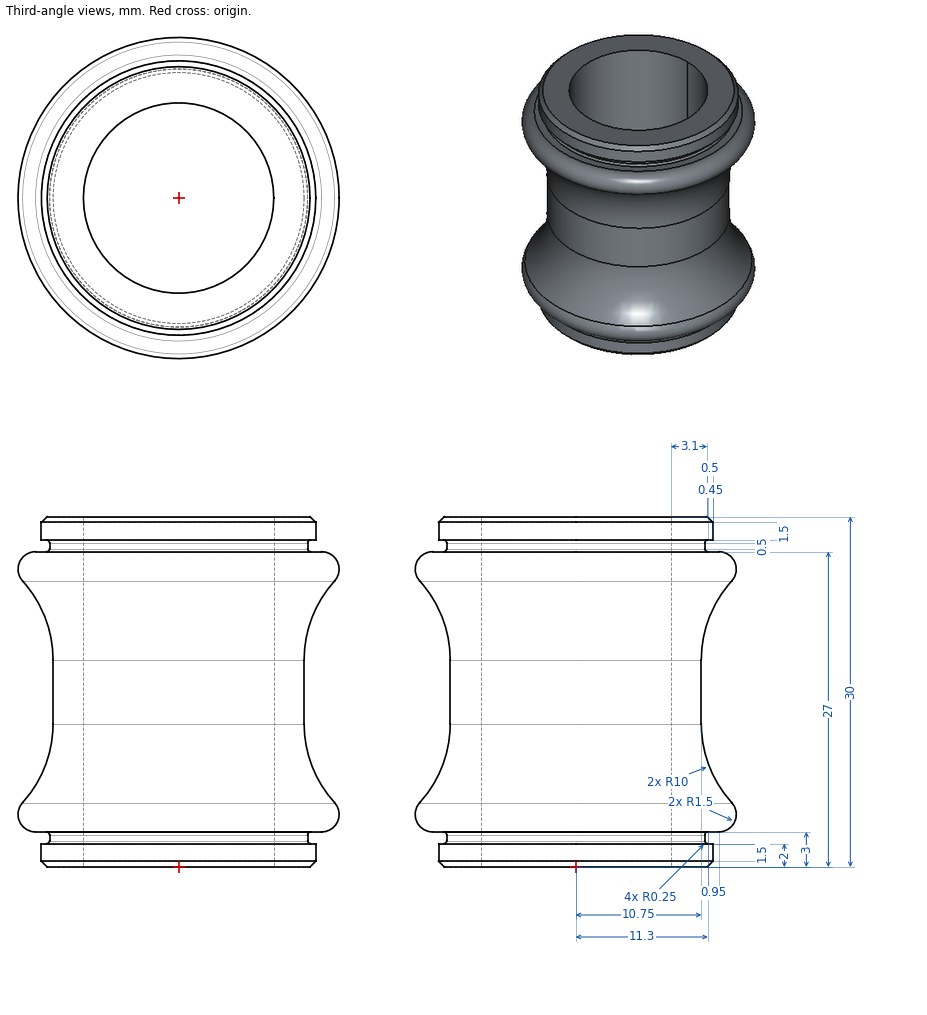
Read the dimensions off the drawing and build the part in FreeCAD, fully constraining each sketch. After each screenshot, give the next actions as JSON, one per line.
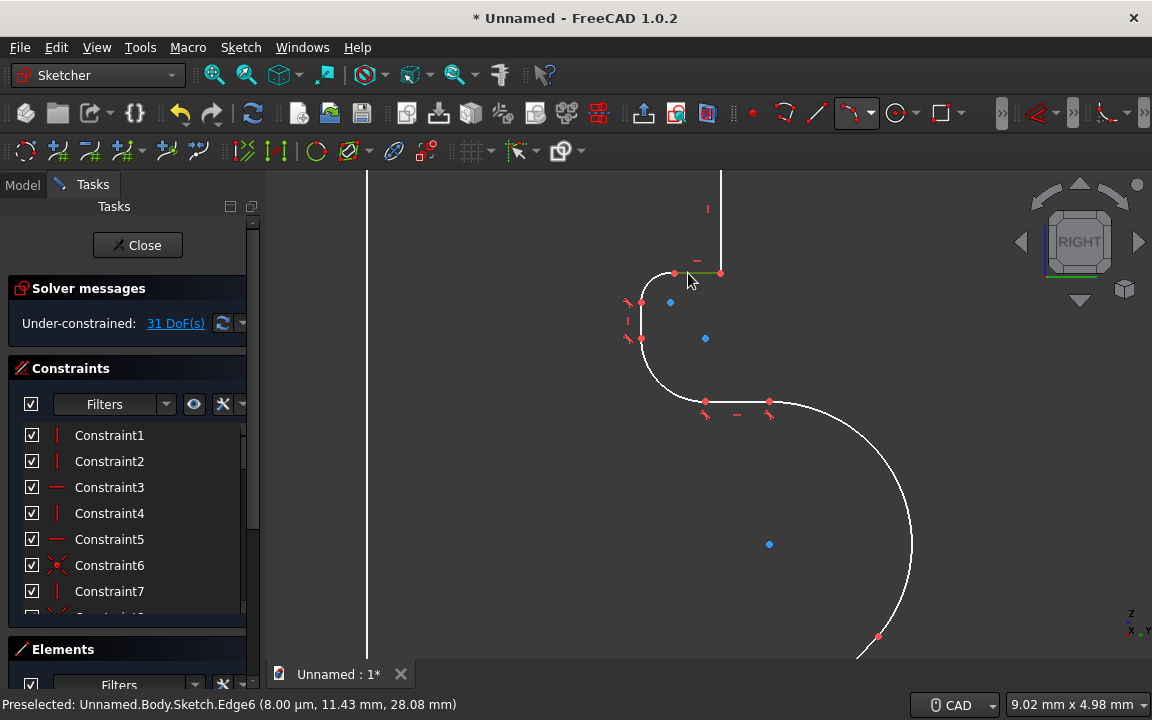
{"action": "left_click", "coordinate": [659, 275]}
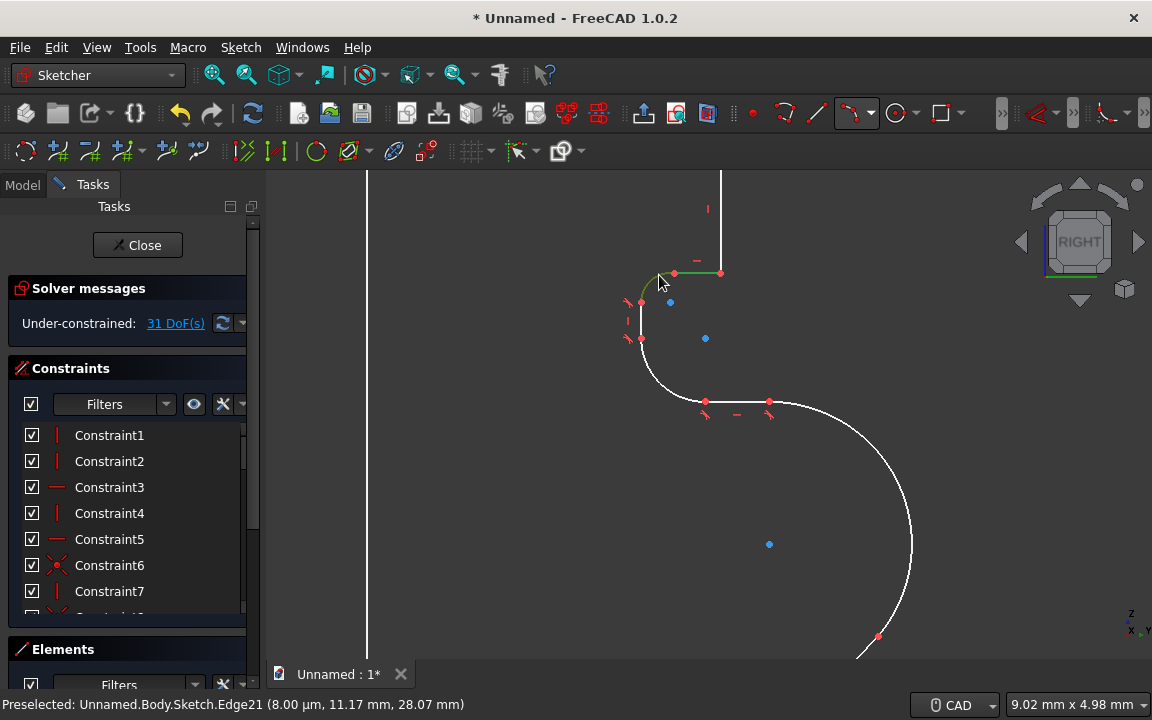
{"action": "key", "text": "t"}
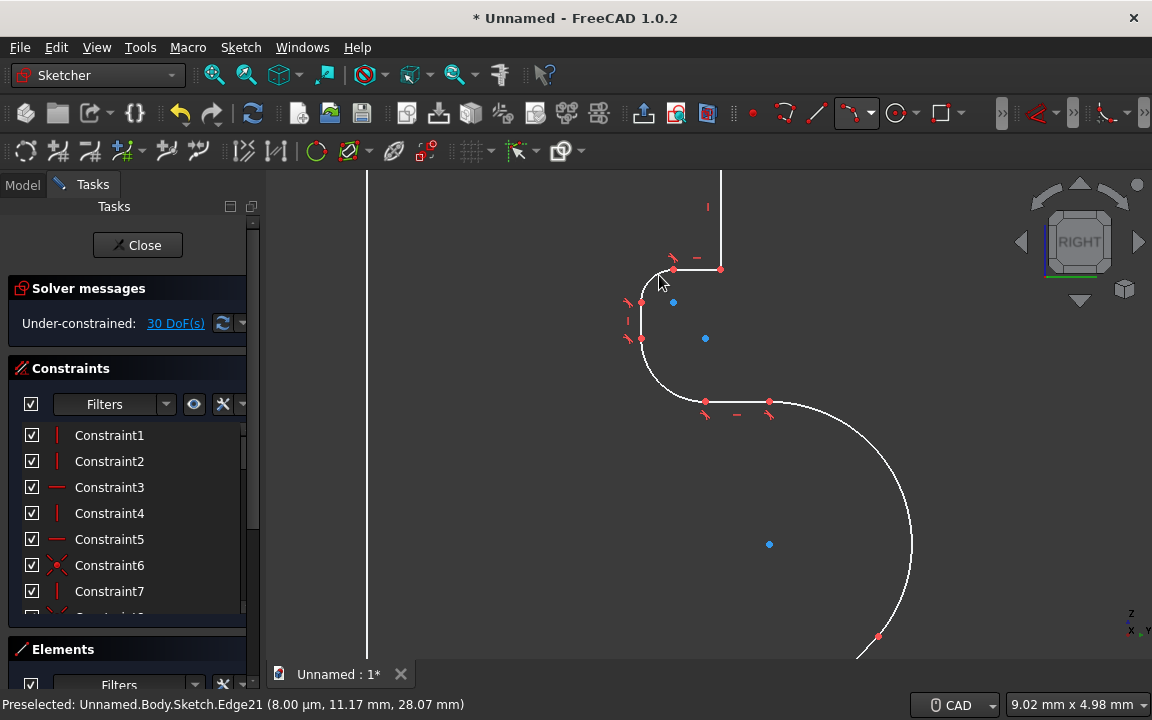
{"action": "scroll", "coordinate": [691, 272], "scroll_direction": "down", "scroll_amount": 11}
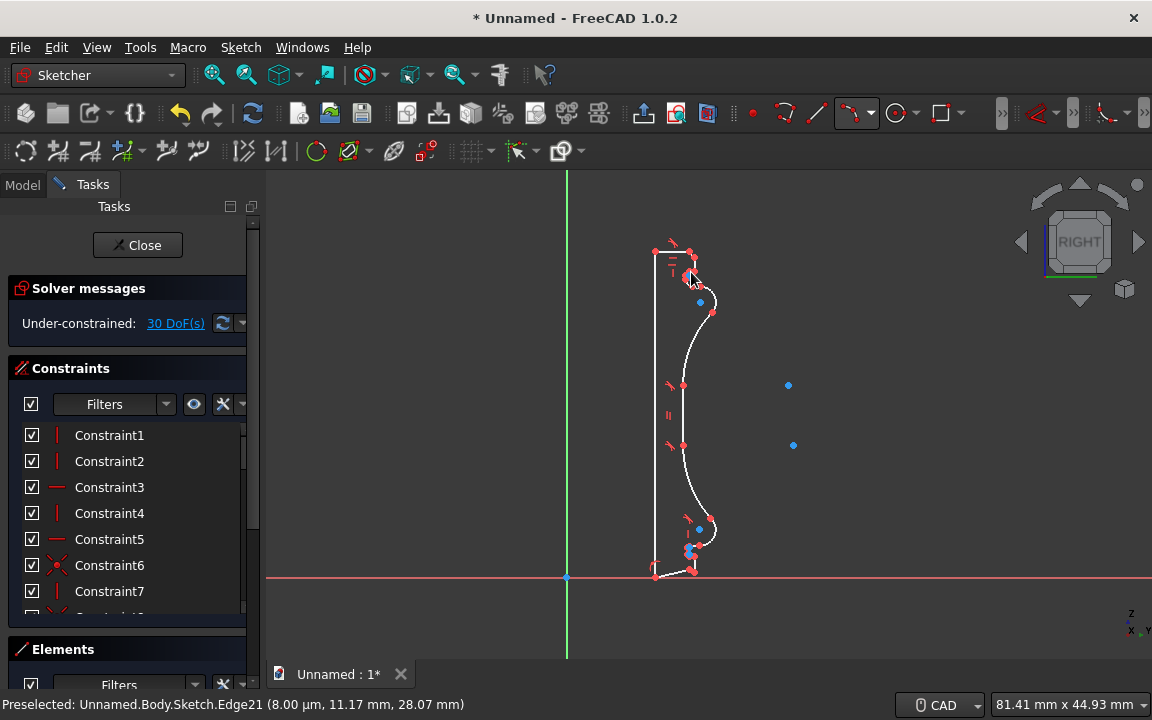
{"action": "scroll", "coordinate": [693, 556], "scroll_direction": "up", "scroll_amount": 12}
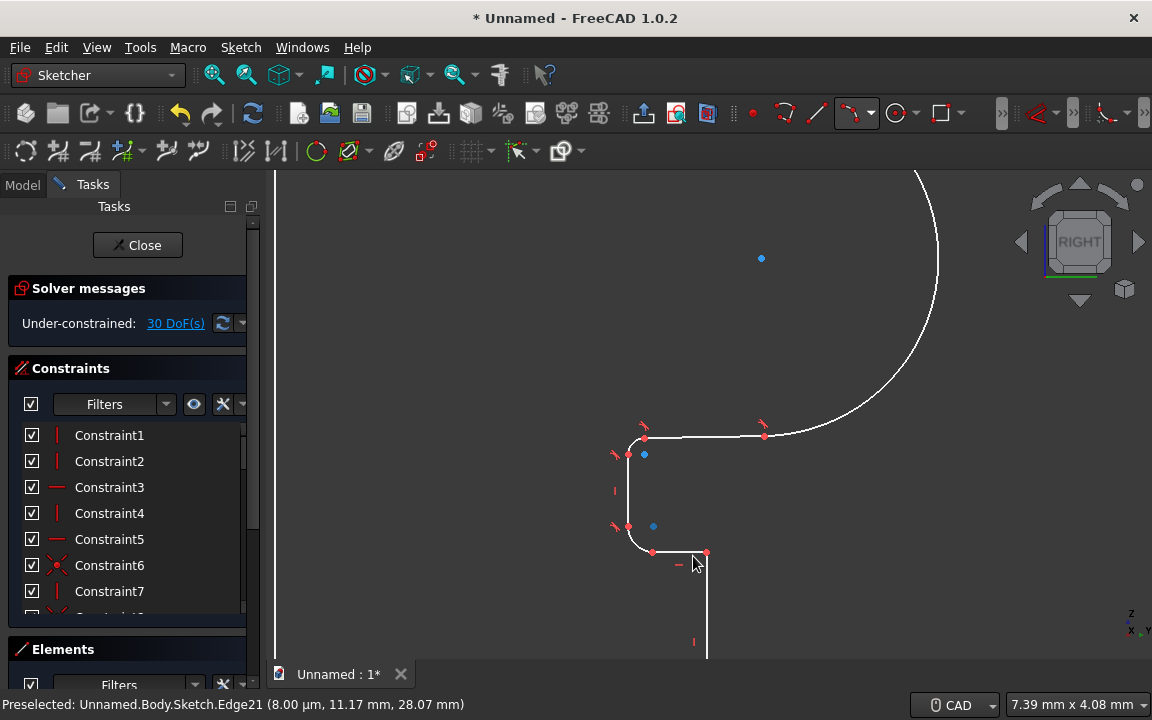
{"action": "left_click", "coordinate": [690, 552]}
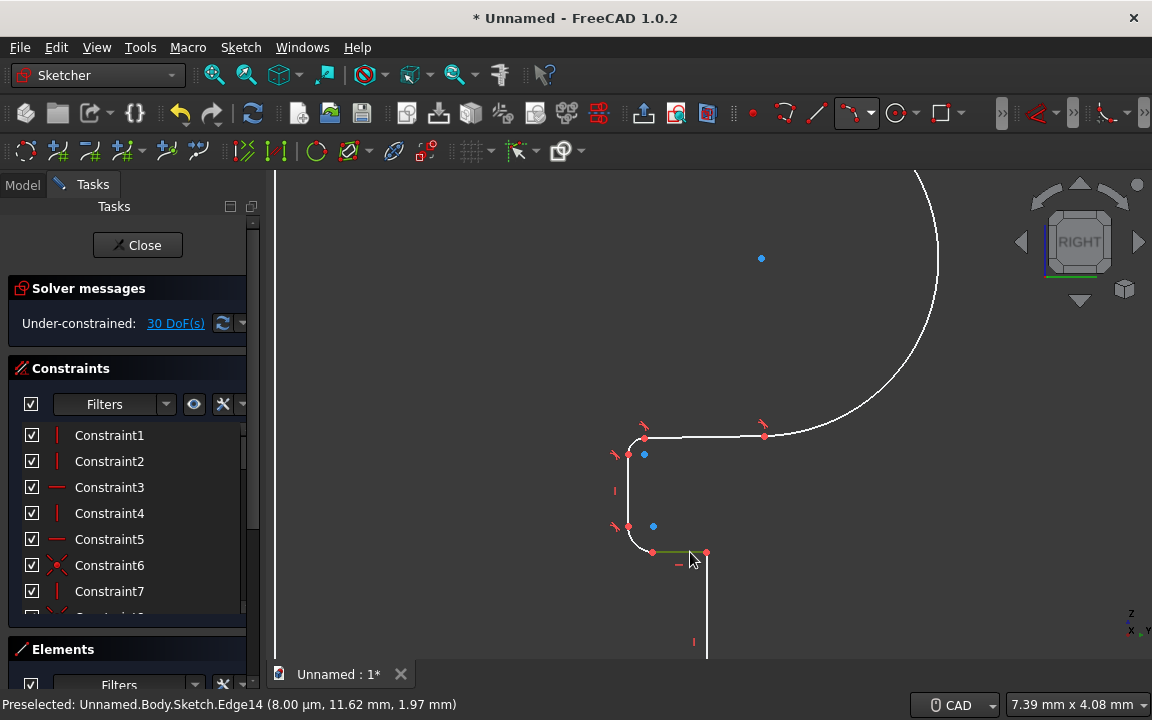
{"action": "left_click", "coordinate": [631, 538]}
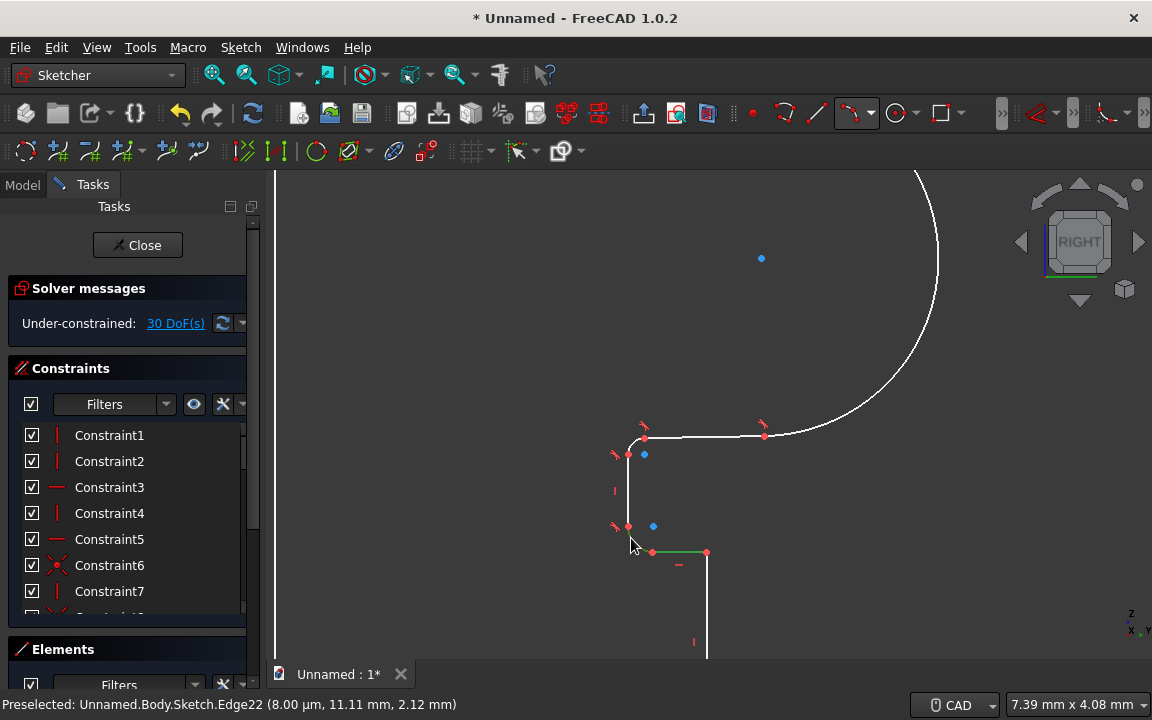
{"action": "key", "text": "t"}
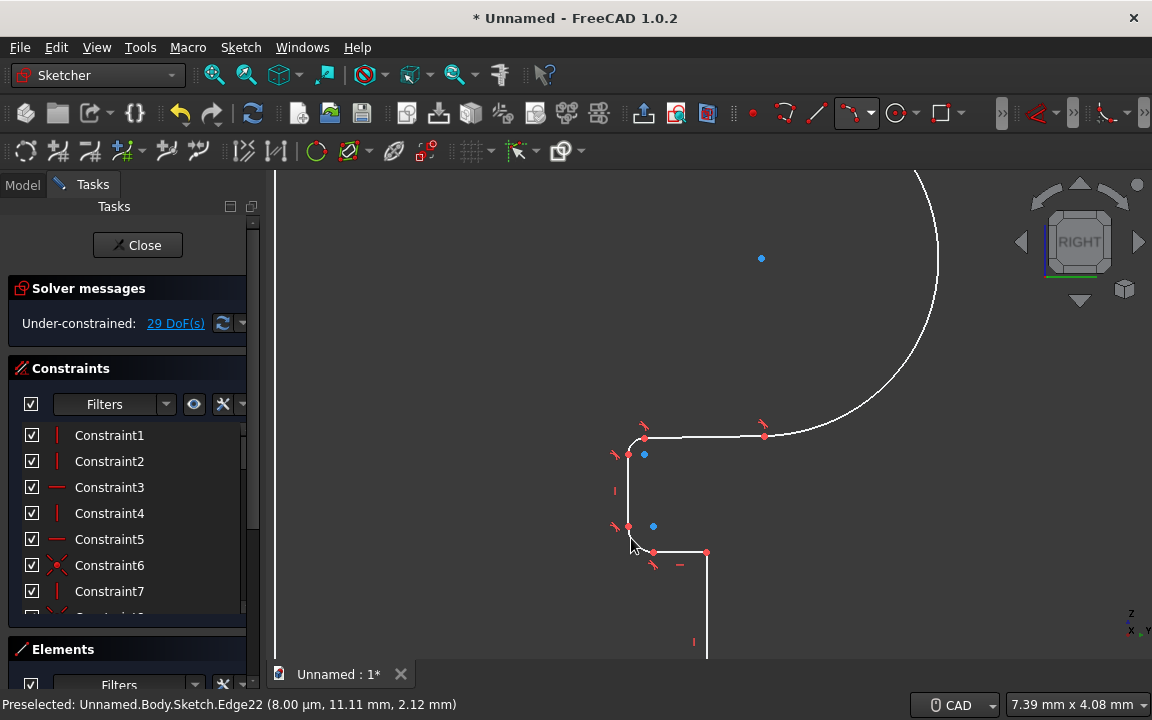
{"action": "scroll", "coordinate": [693, 557], "scroll_direction": "down", "scroll_amount": 12}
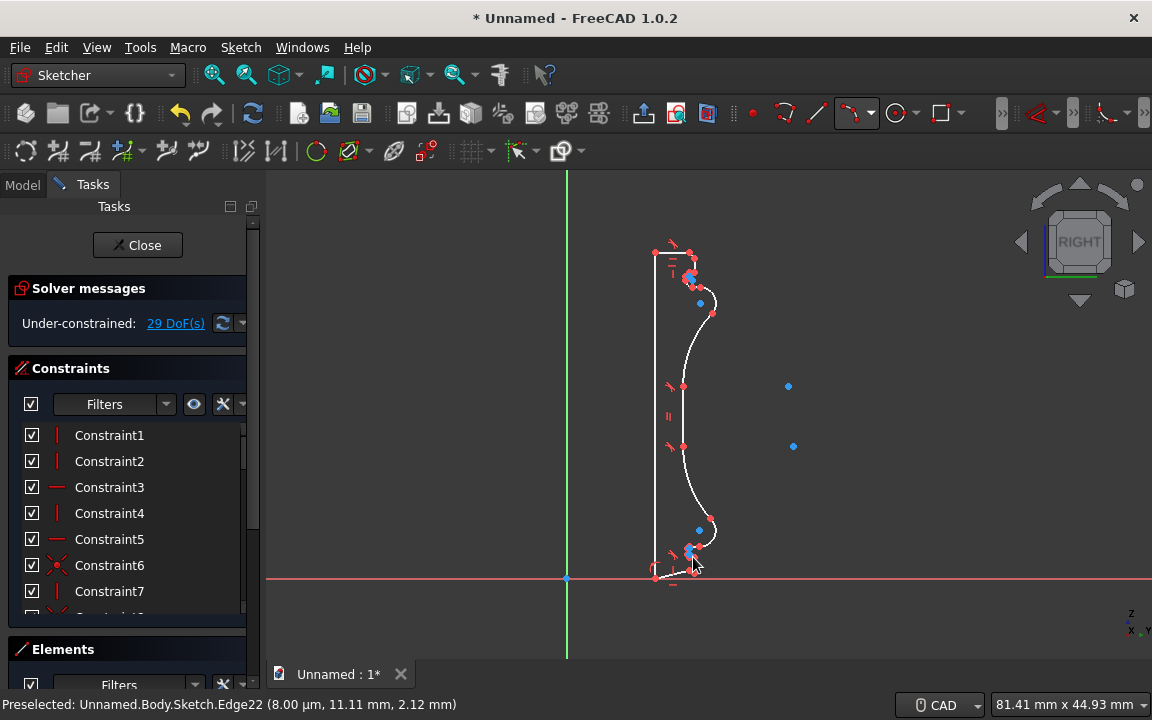
{"action": "scroll", "coordinate": [710, 543], "scroll_direction": "up", "scroll_amount": 2}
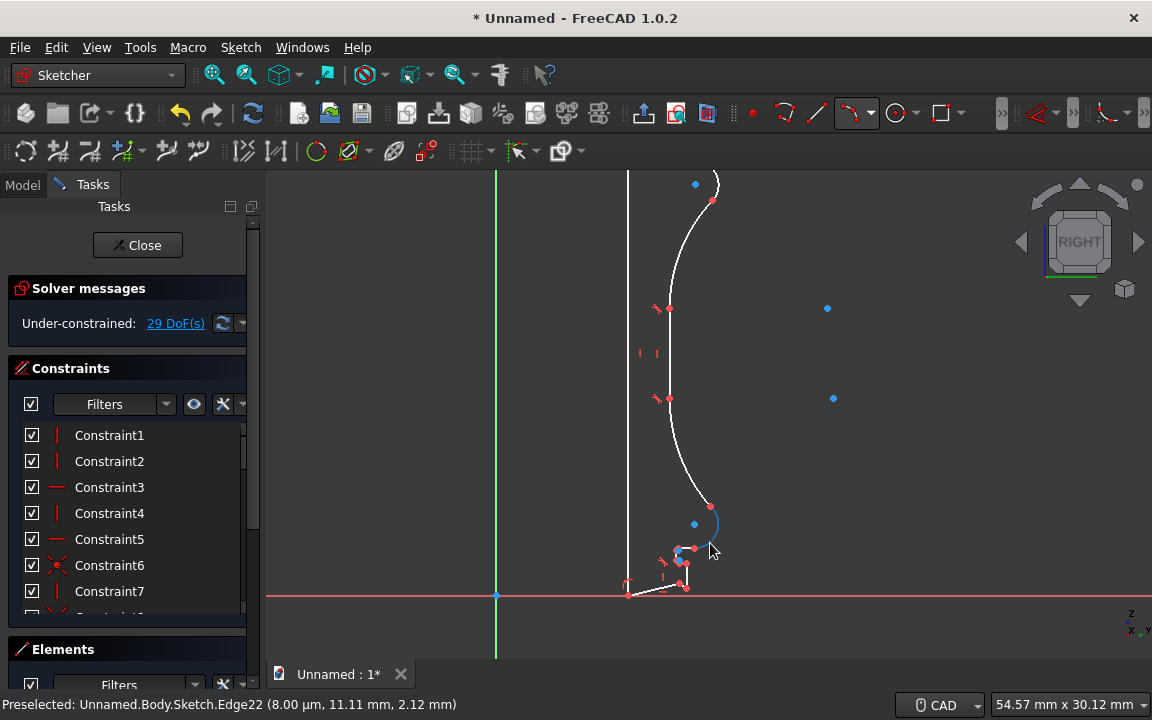
{"action": "left_click", "coordinate": [710, 542]}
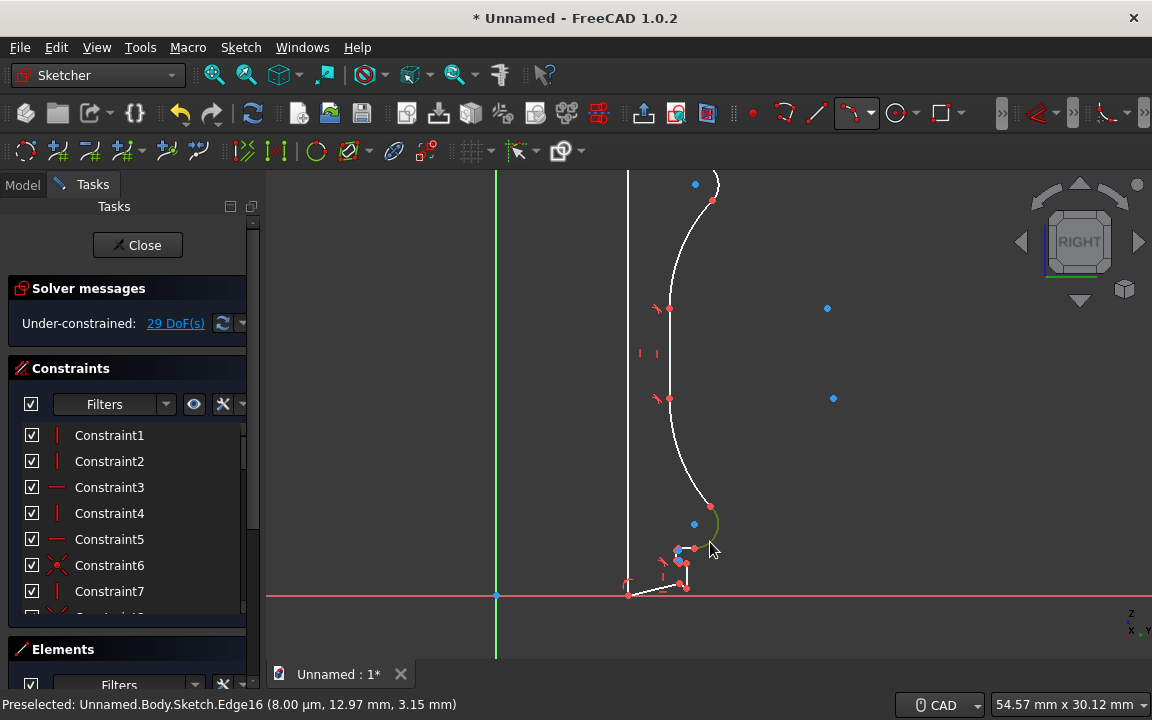
{"action": "left_click", "coordinate": [674, 434]}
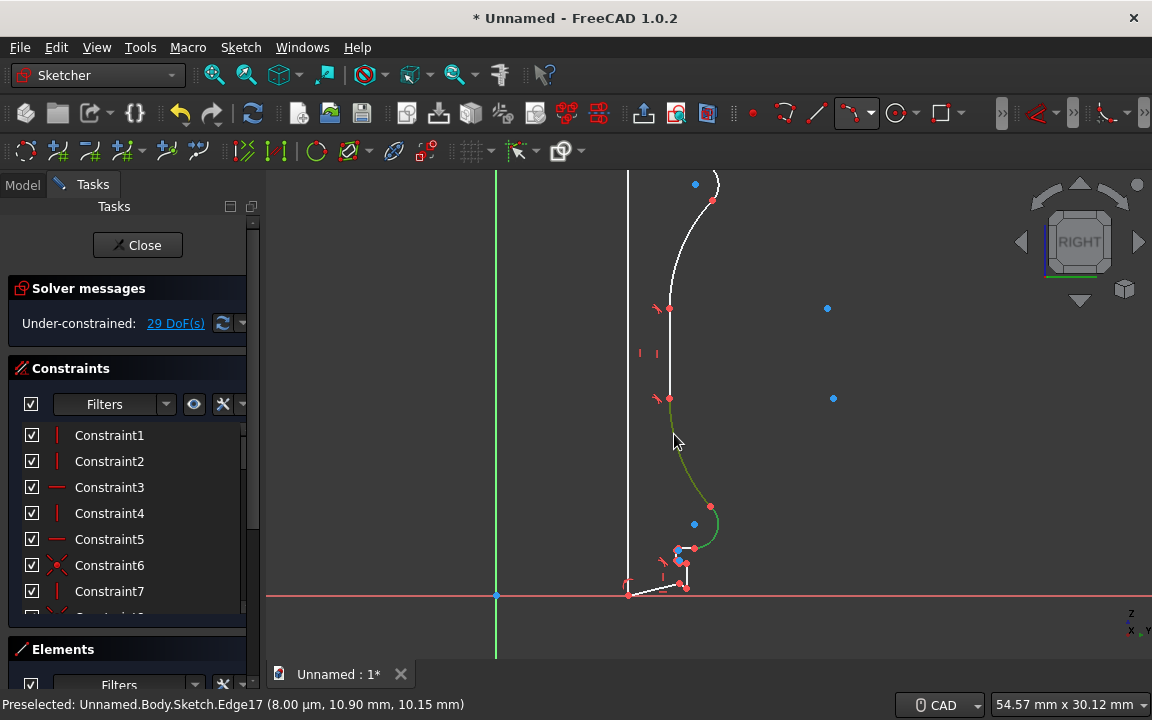
{"action": "key", "text": "t"}